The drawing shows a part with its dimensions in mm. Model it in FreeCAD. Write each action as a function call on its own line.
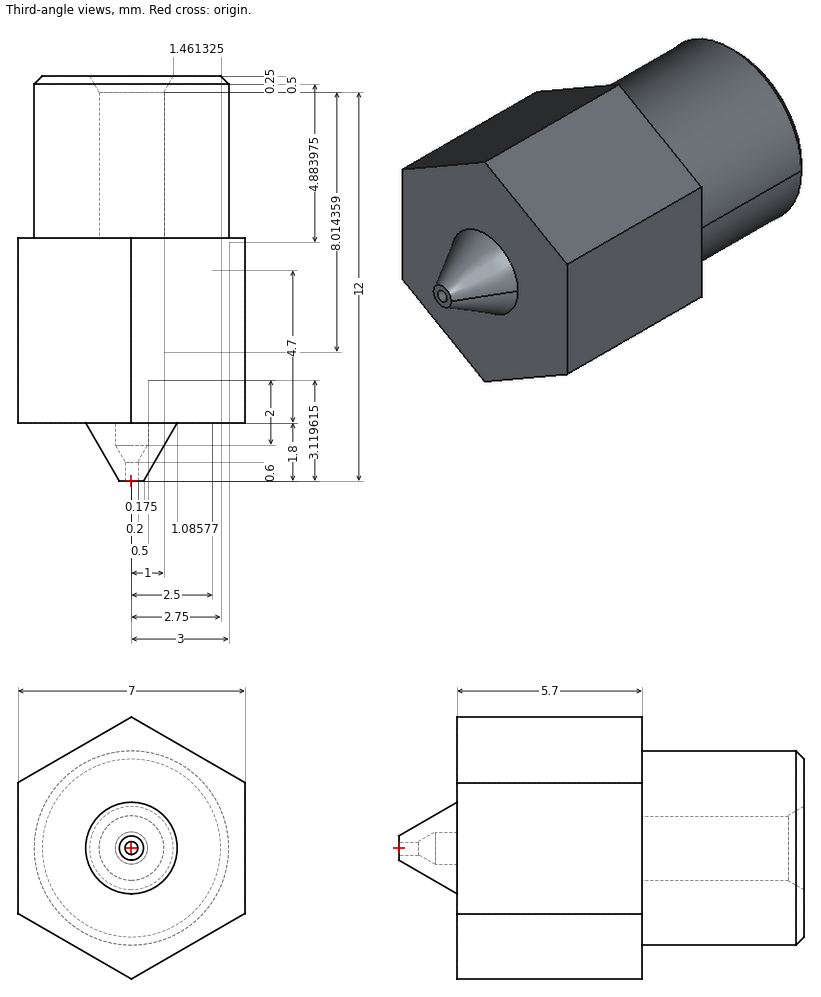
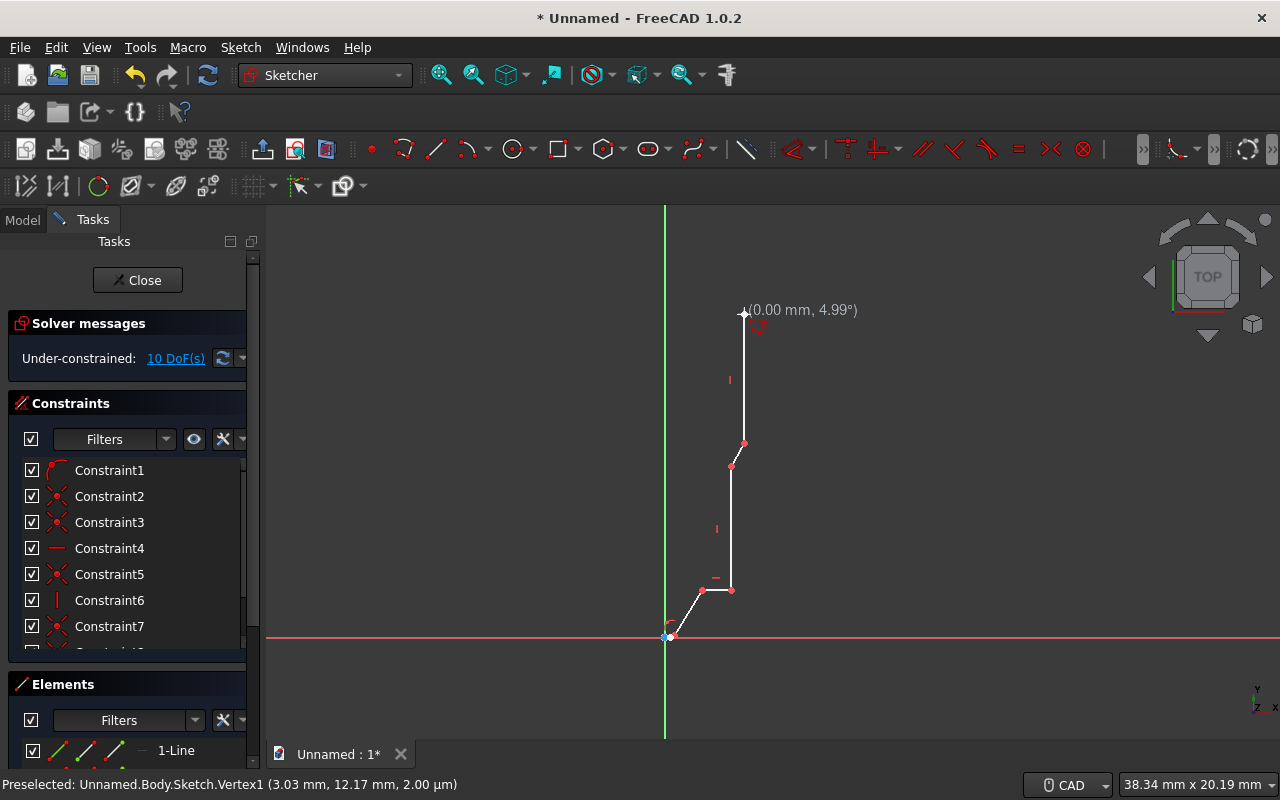
scroll(738, 307, up, 3)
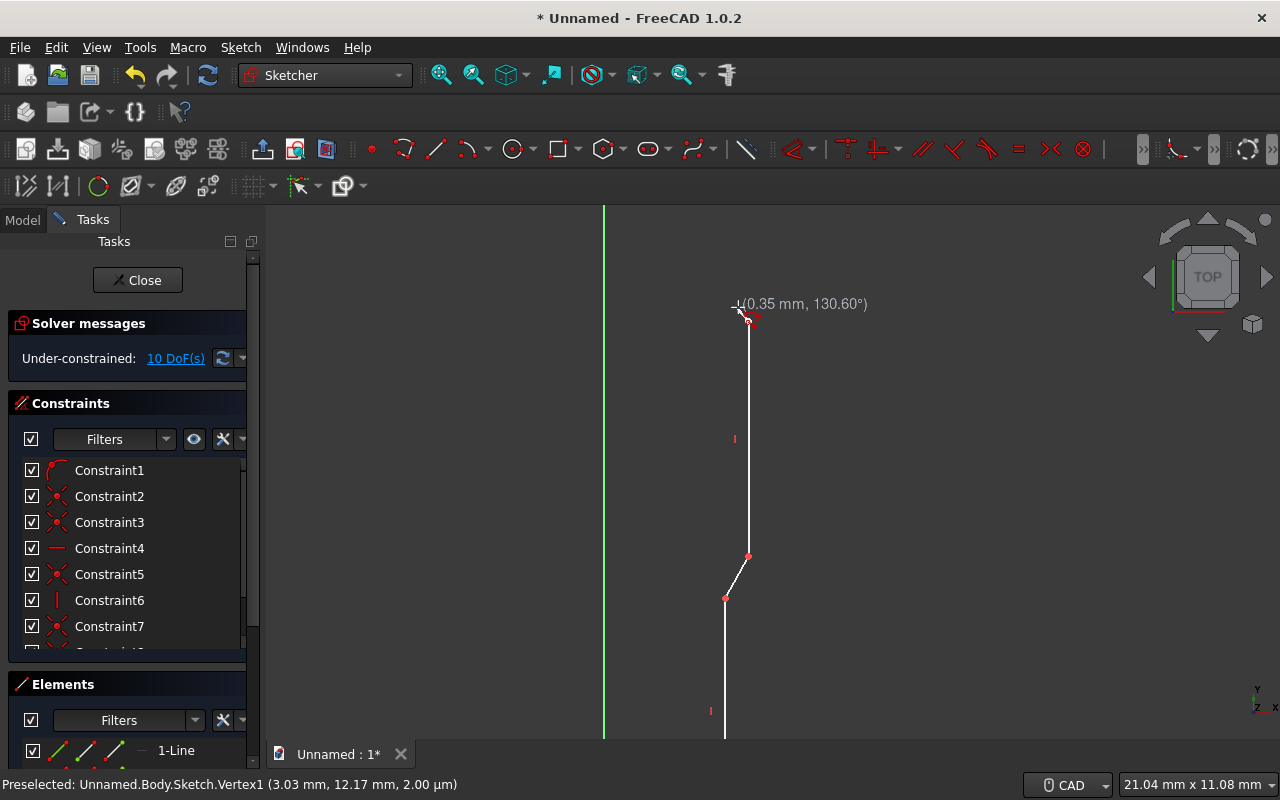
click(737, 307)
click(666, 307)
click(653, 331)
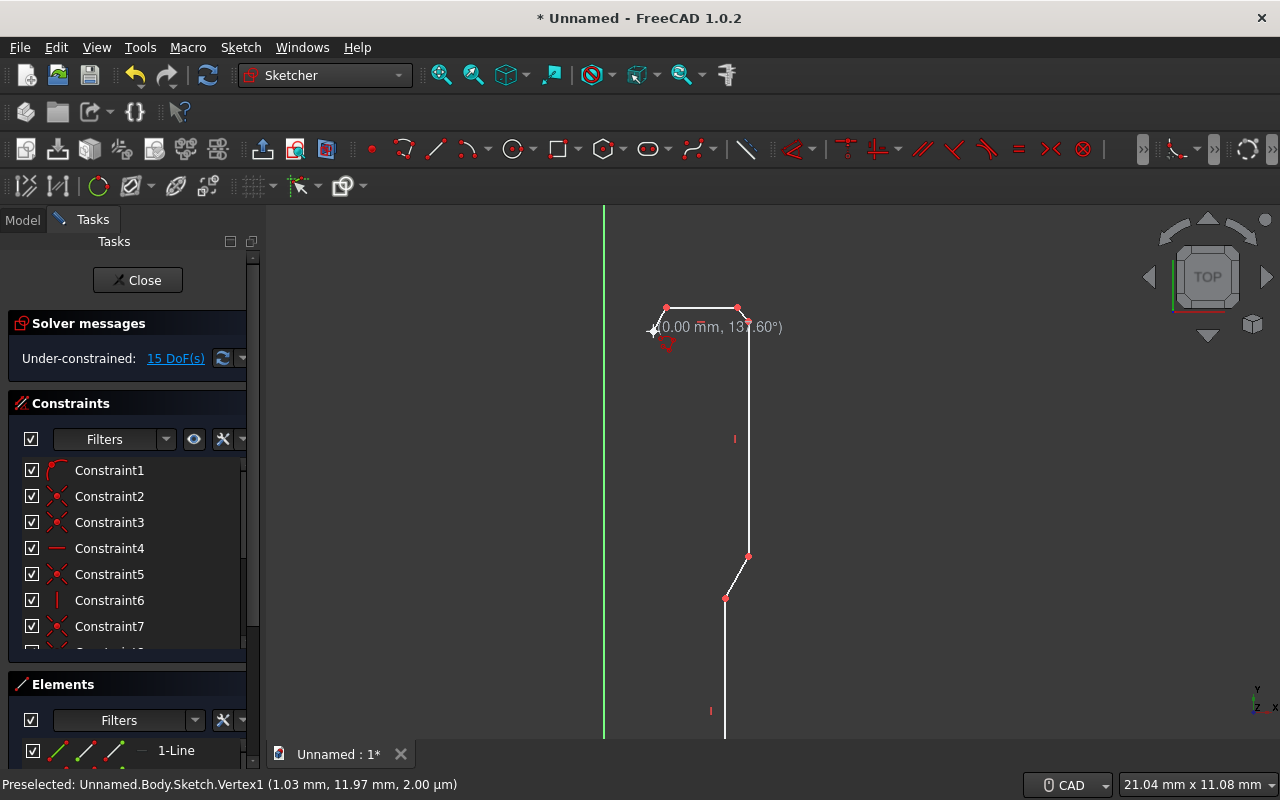
scroll(738, 306, down, 3)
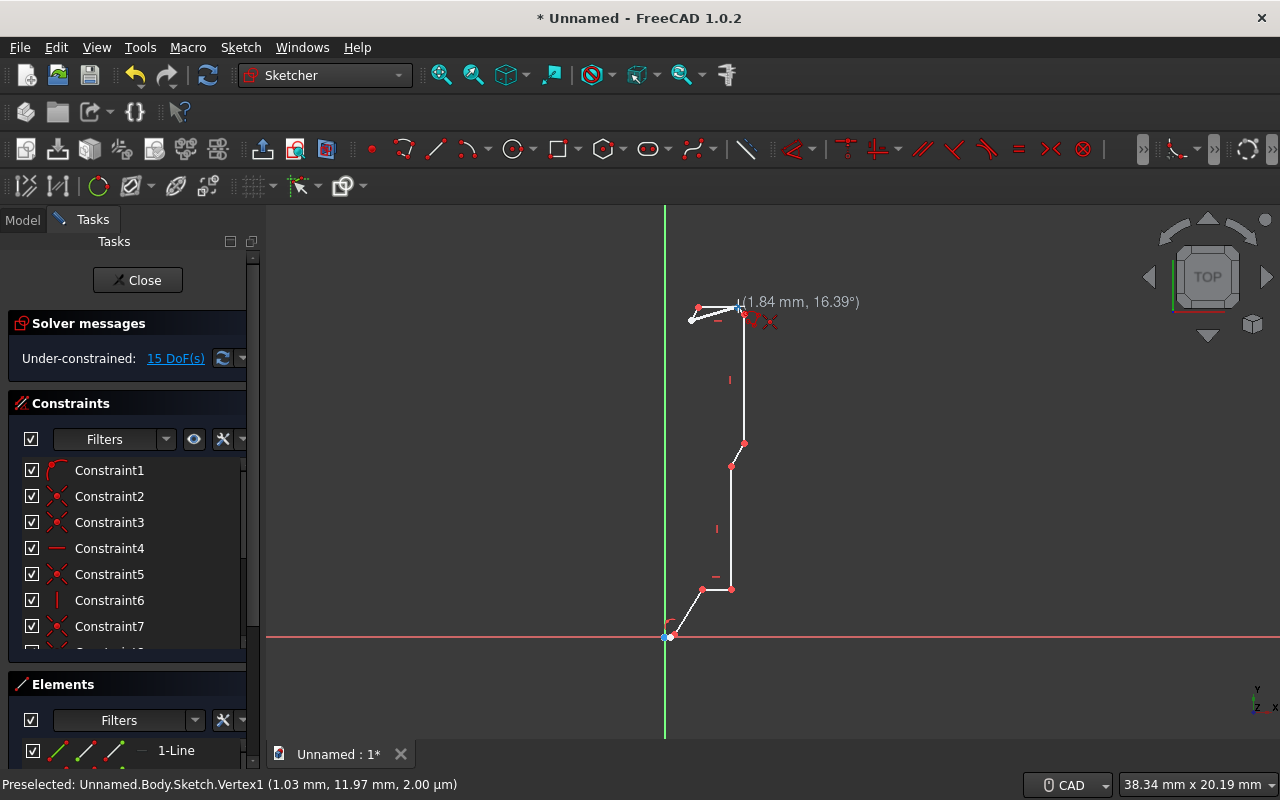
click(692, 532)
click(678, 555)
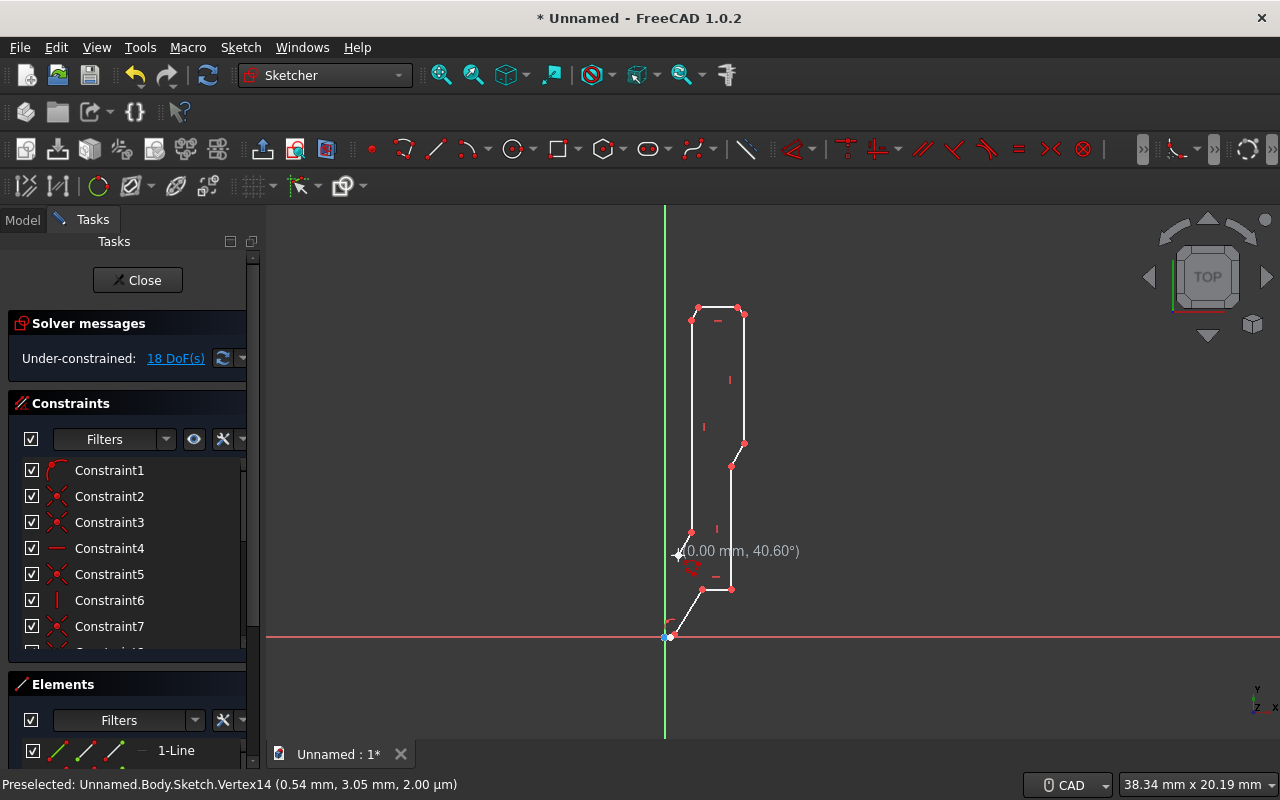
scroll(678, 608, up, 2)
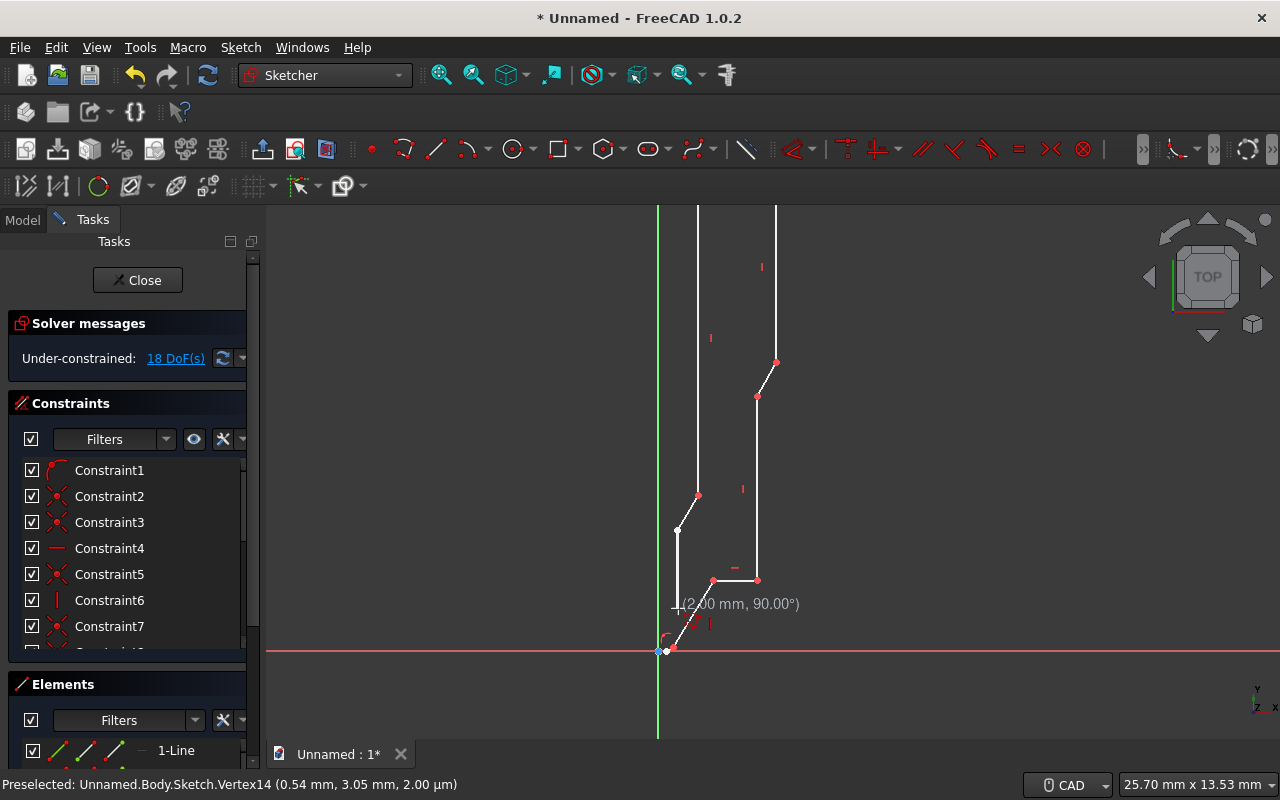
click(678, 607)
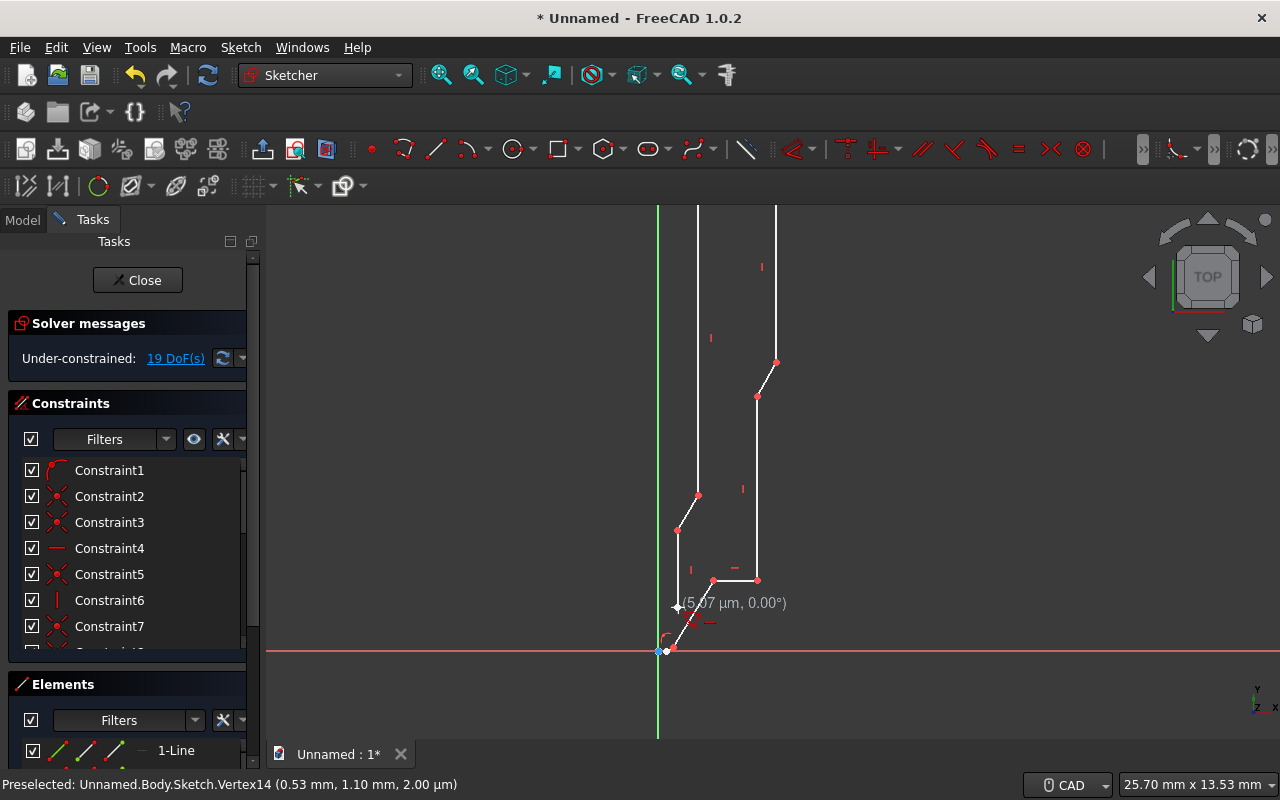
scroll(666, 628, up, 4)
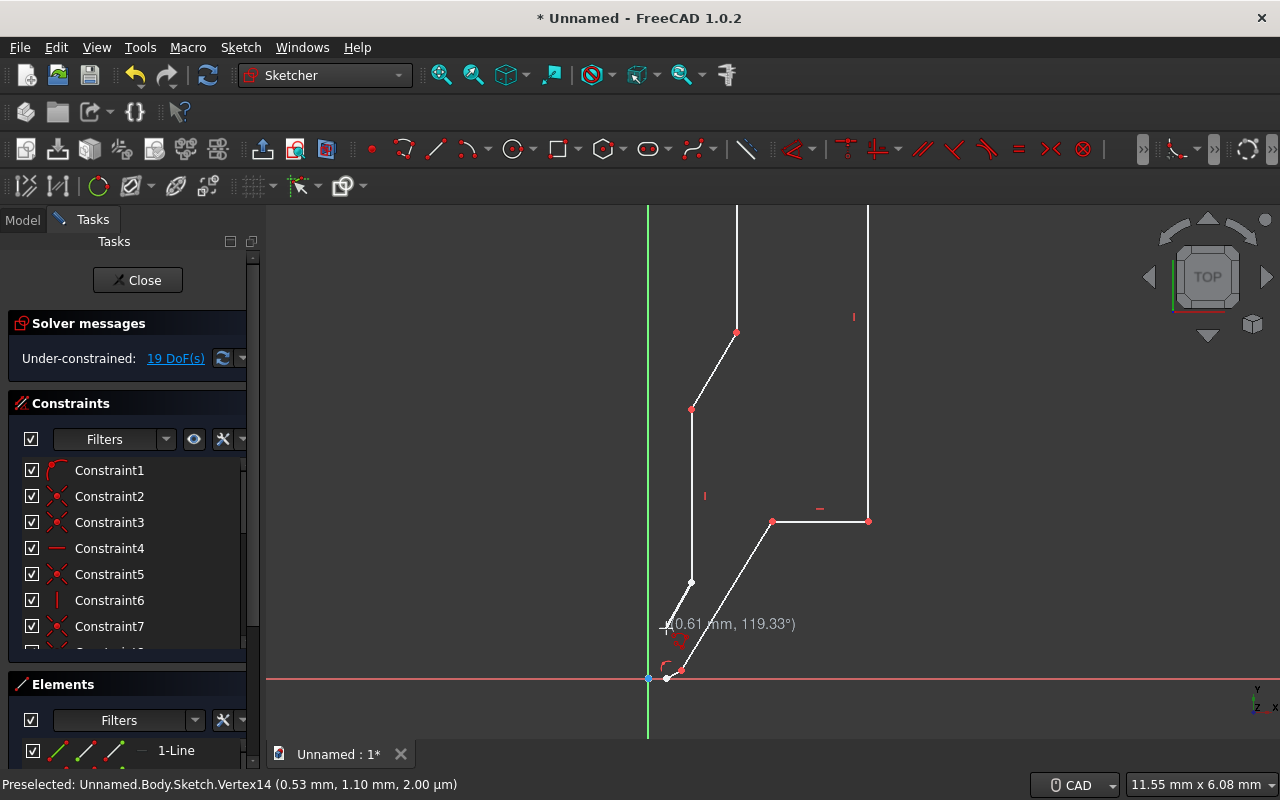
click(666, 626)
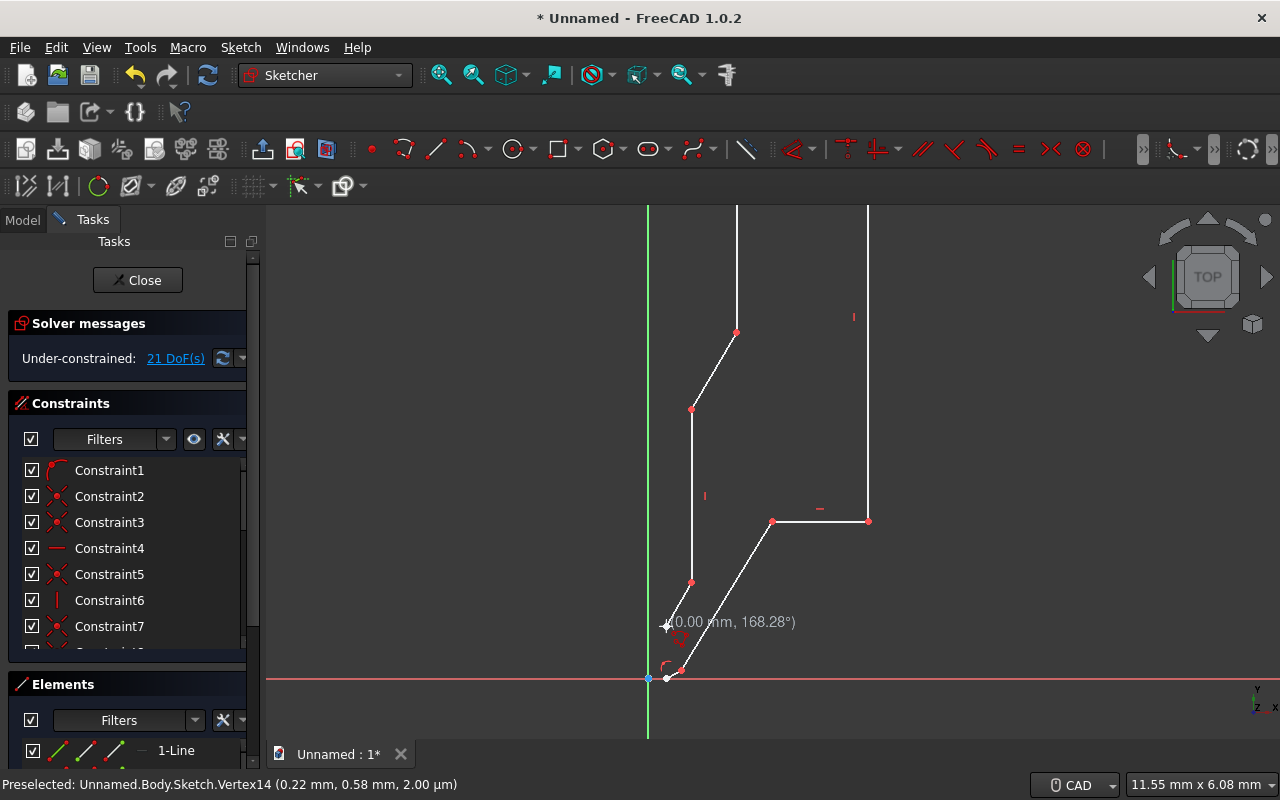
scroll(666, 679, up, 4)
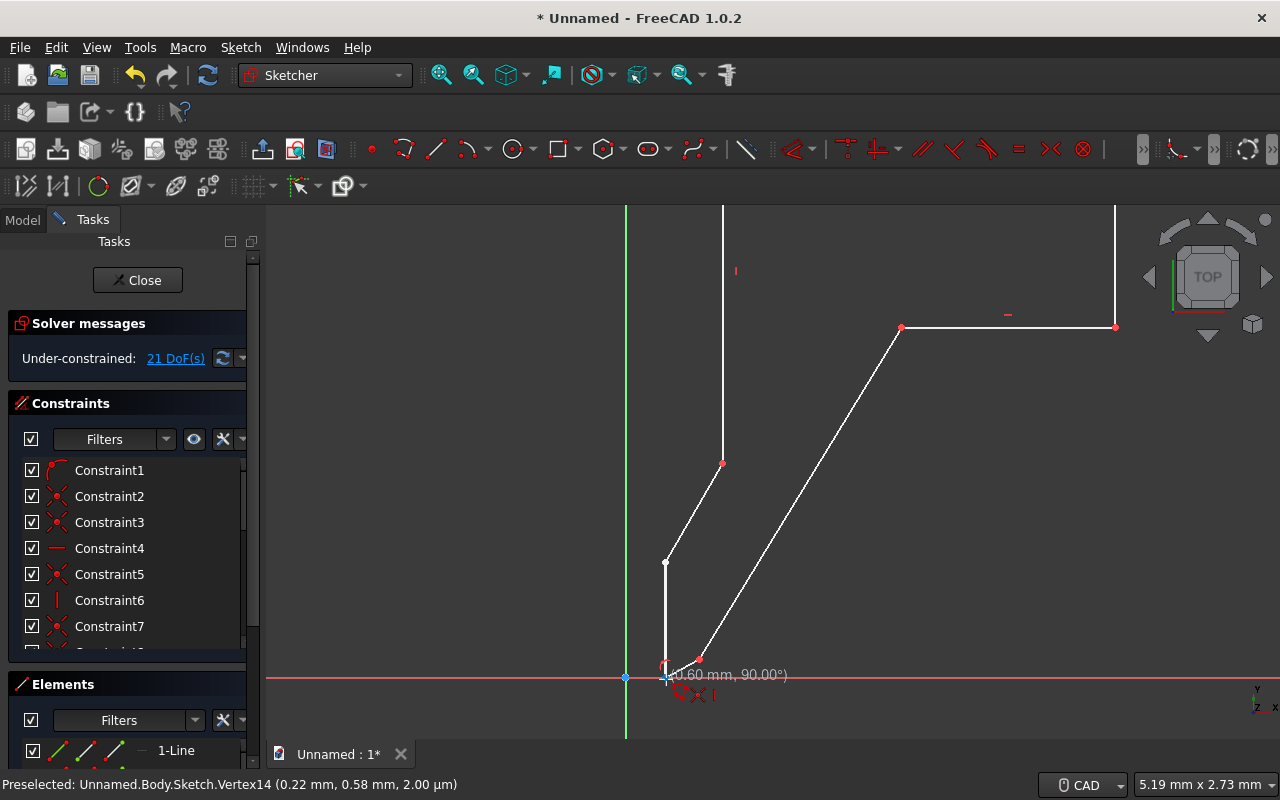
click(666, 678)
key(Escape)
key(Escape)